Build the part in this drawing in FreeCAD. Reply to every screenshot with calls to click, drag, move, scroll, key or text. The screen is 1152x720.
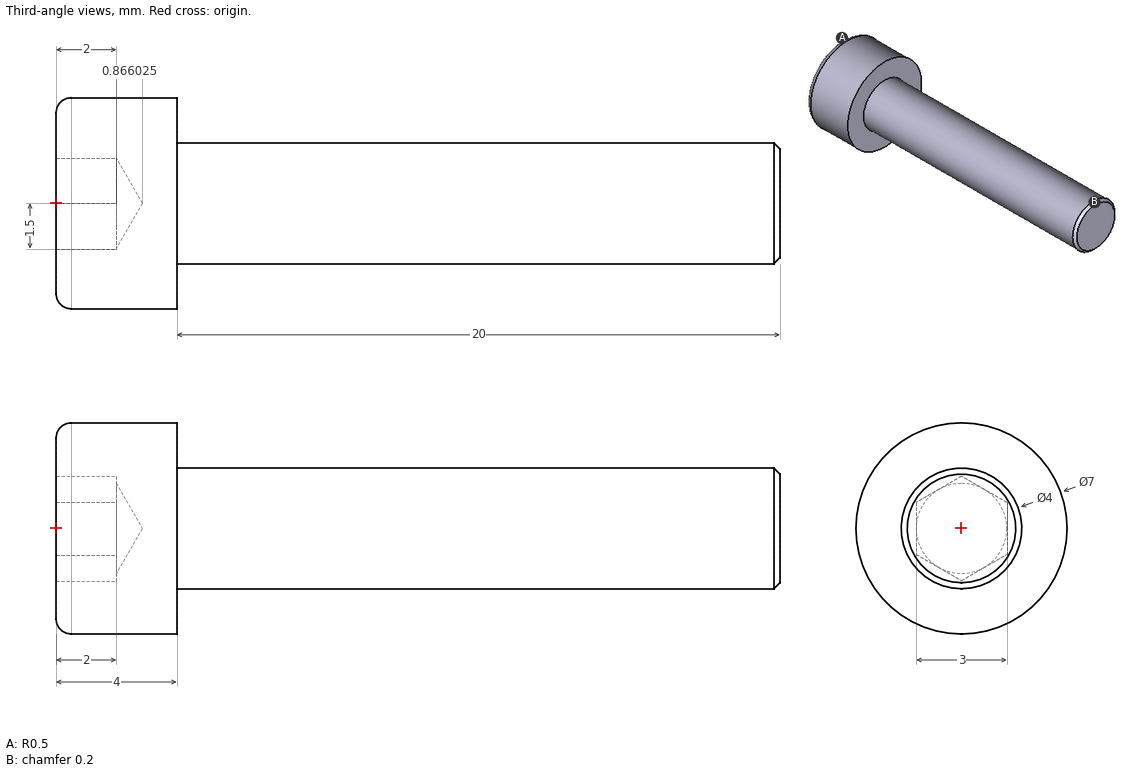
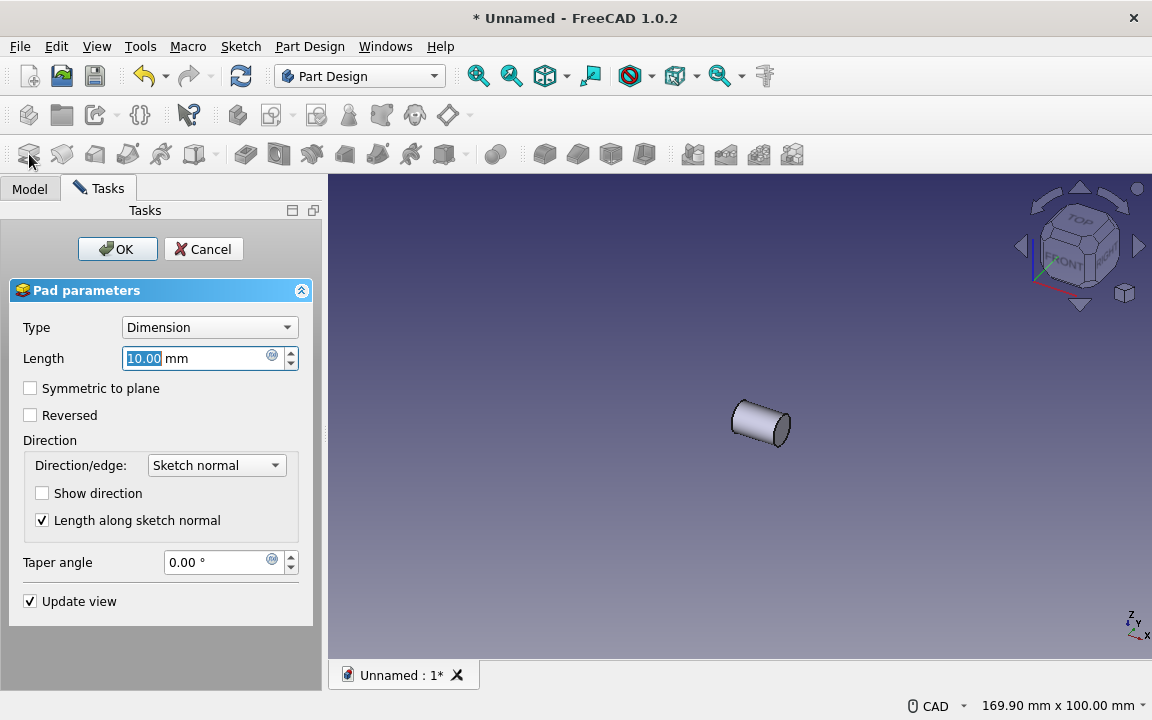
text(4)
key(Tab)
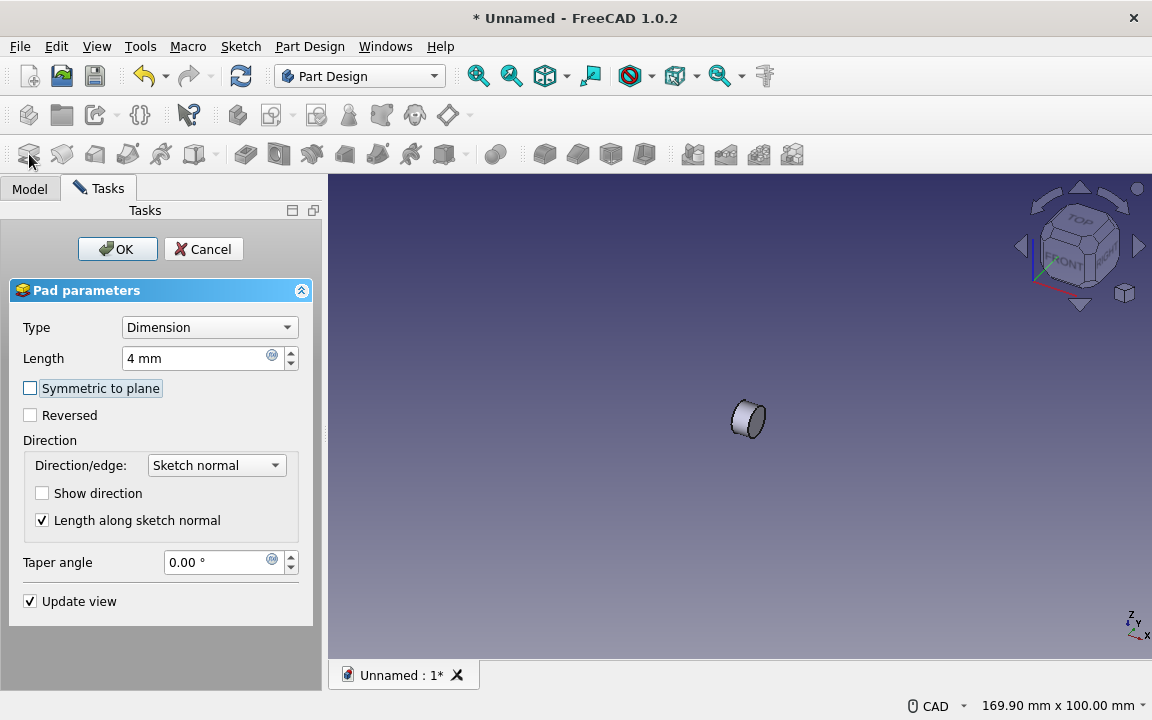
click(118, 249)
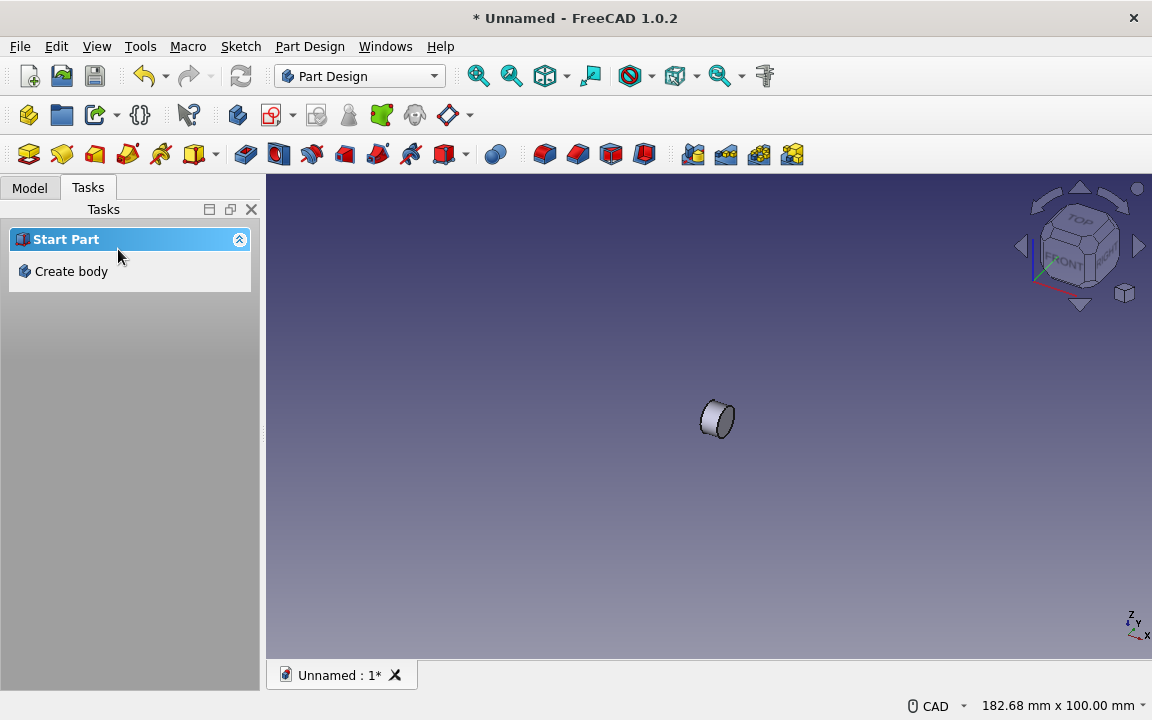
click(479, 76)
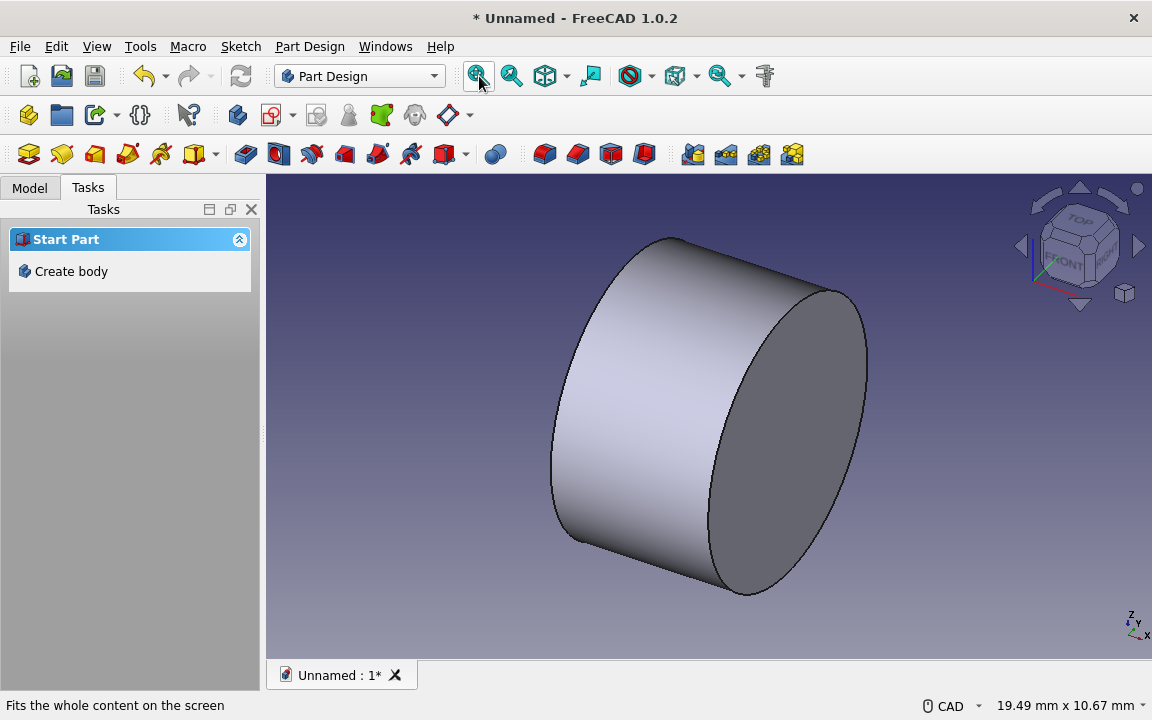
click(788, 442)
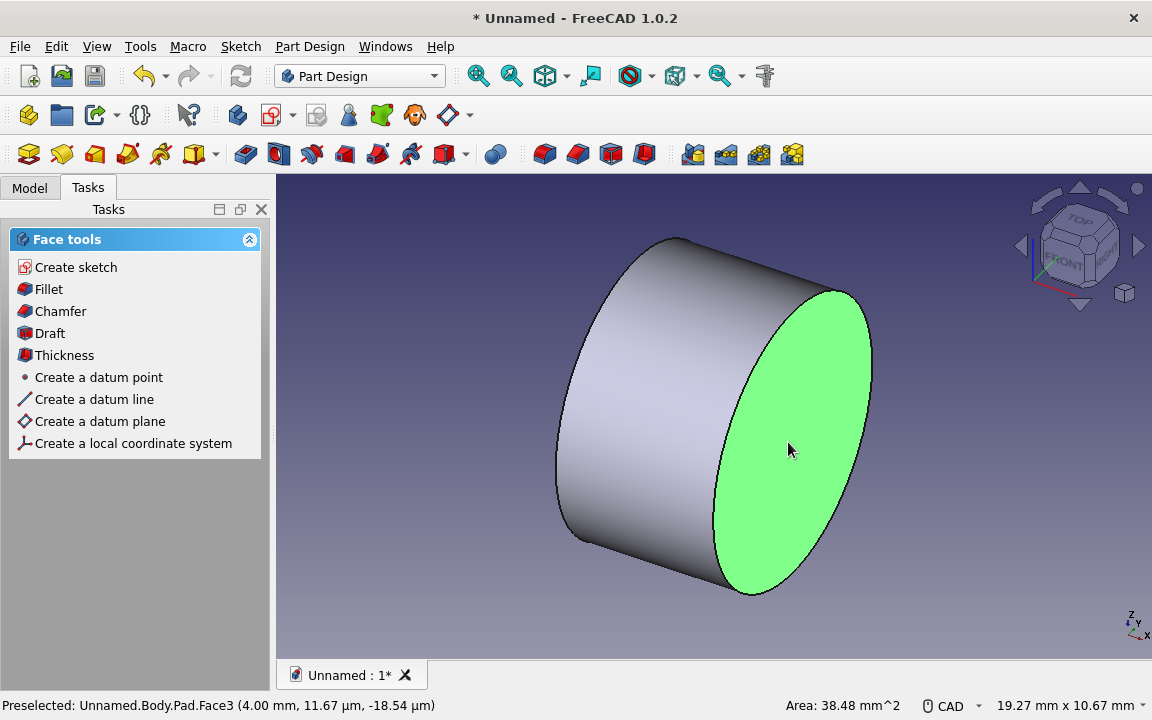
click(270, 116)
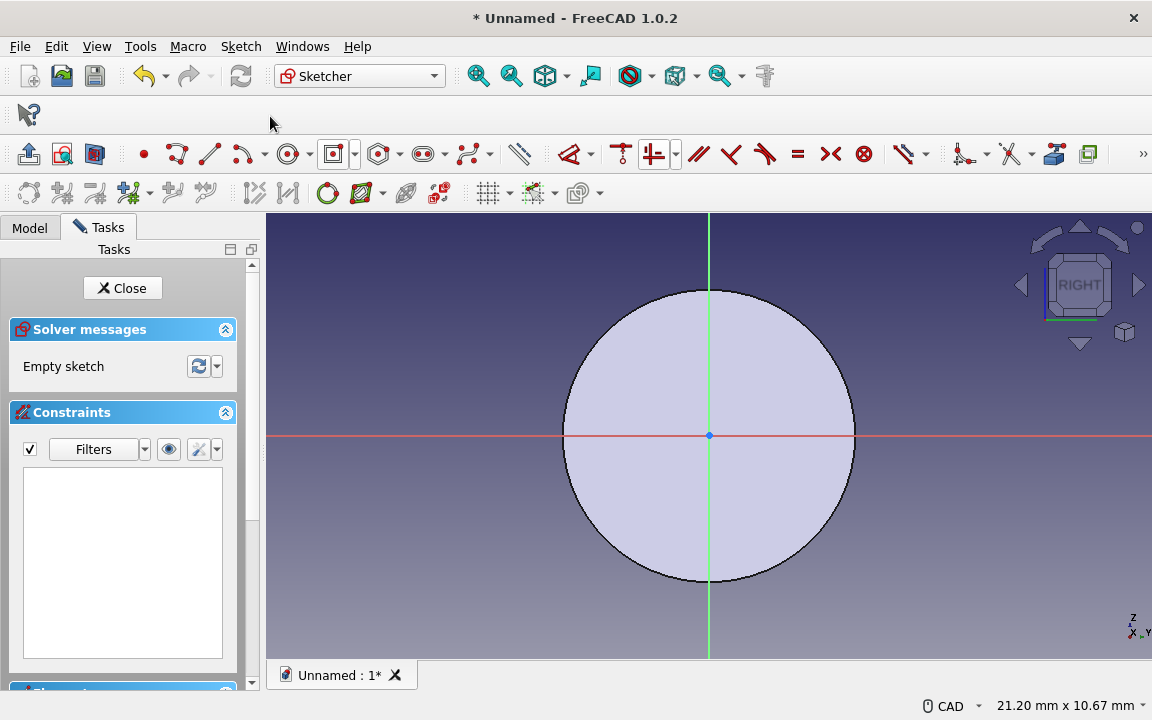
scroll(848, 436, up, 2)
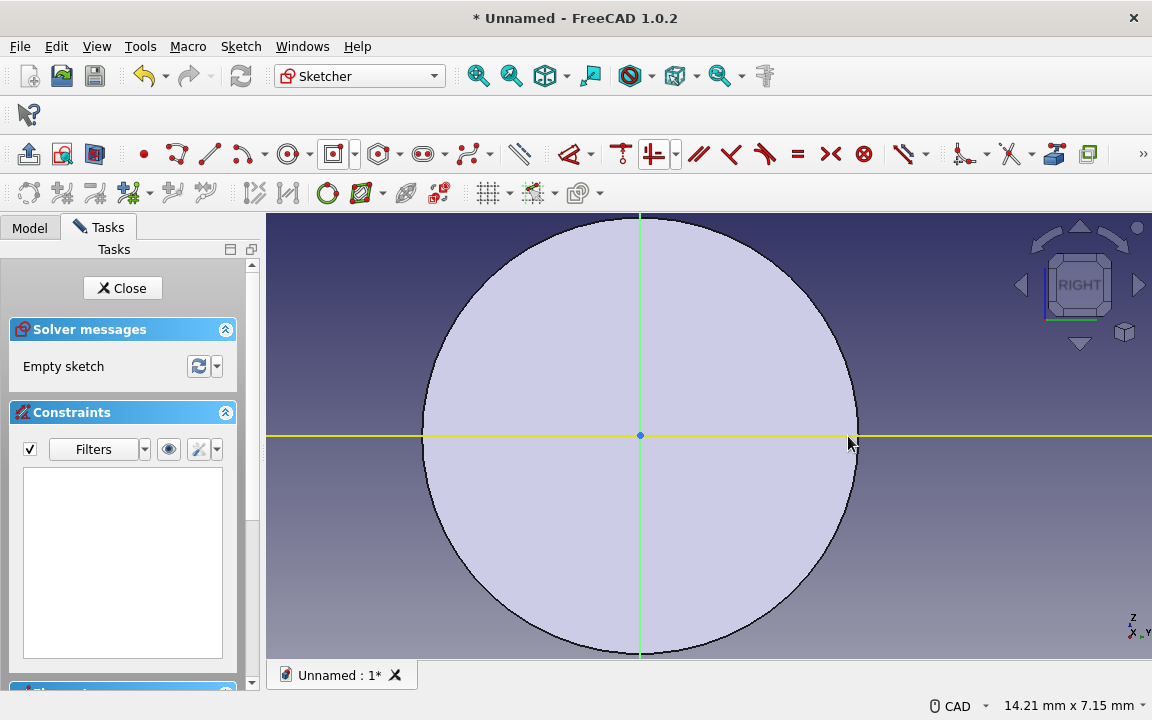
click(288, 154)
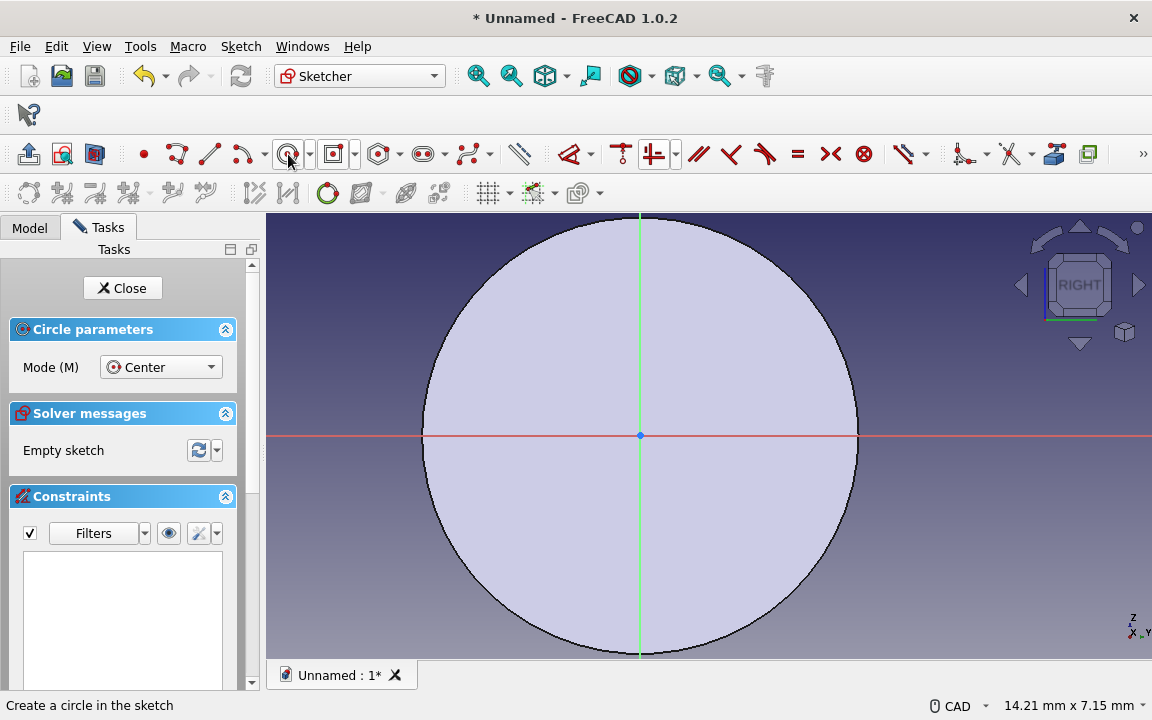
click(640, 436)
click(729, 348)
key(Escape)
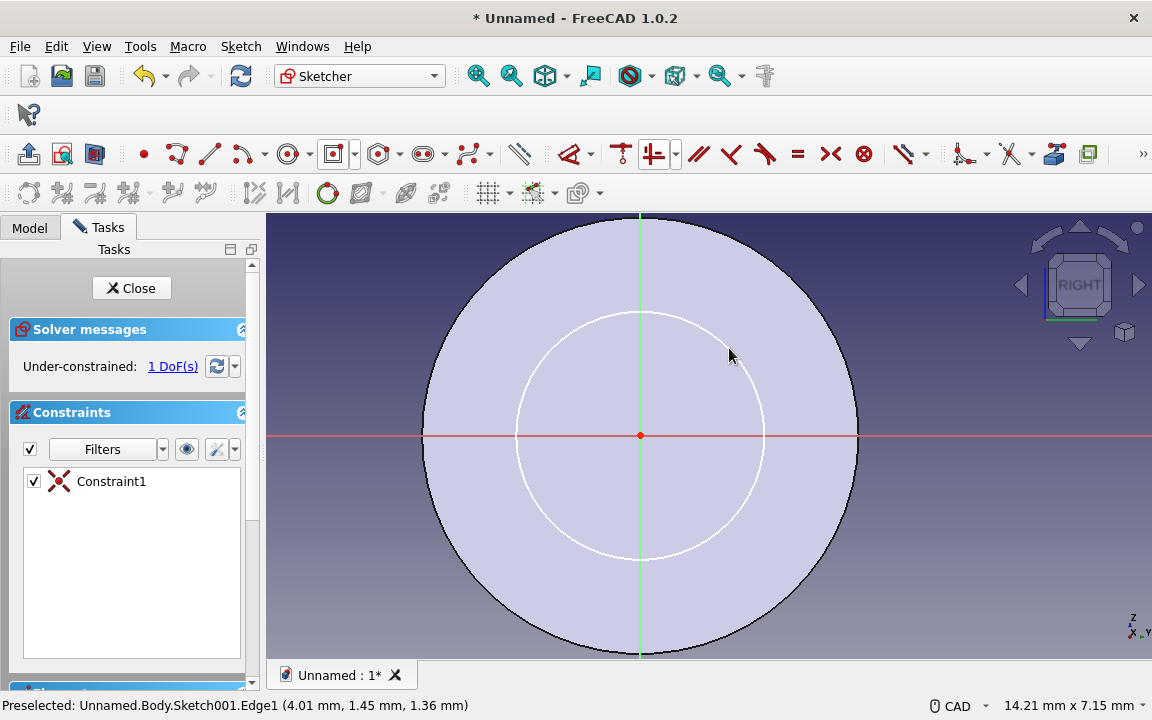
click(568, 154)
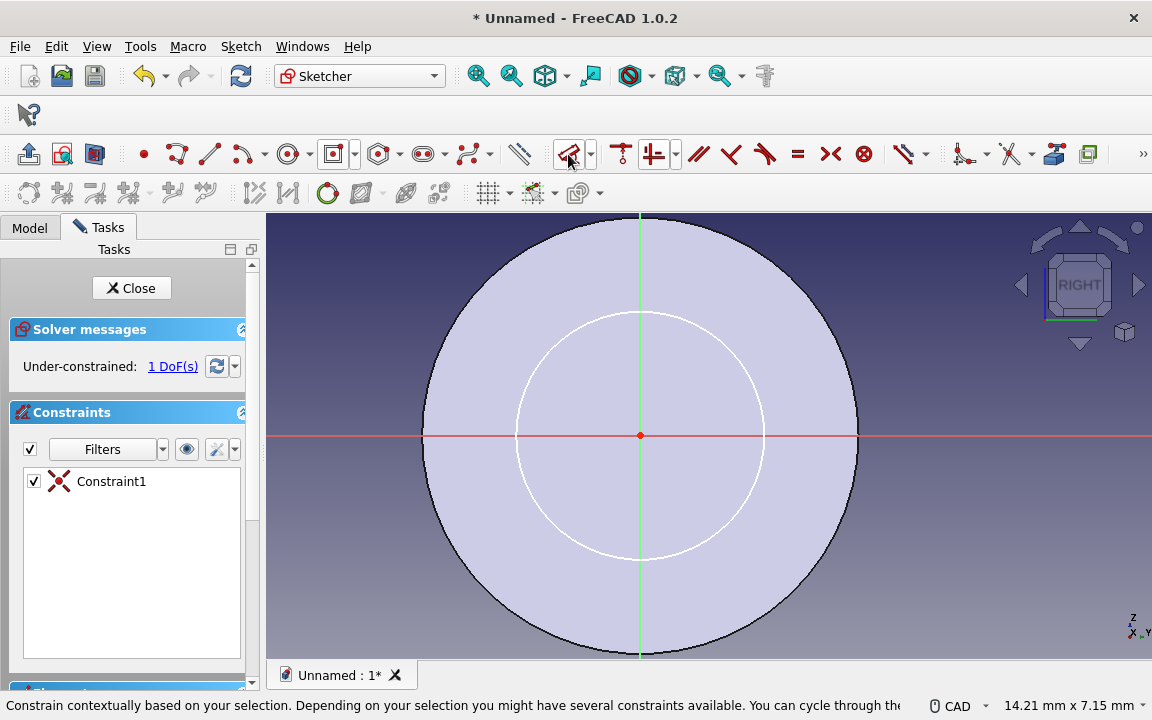
click(728, 348)
click(751, 325)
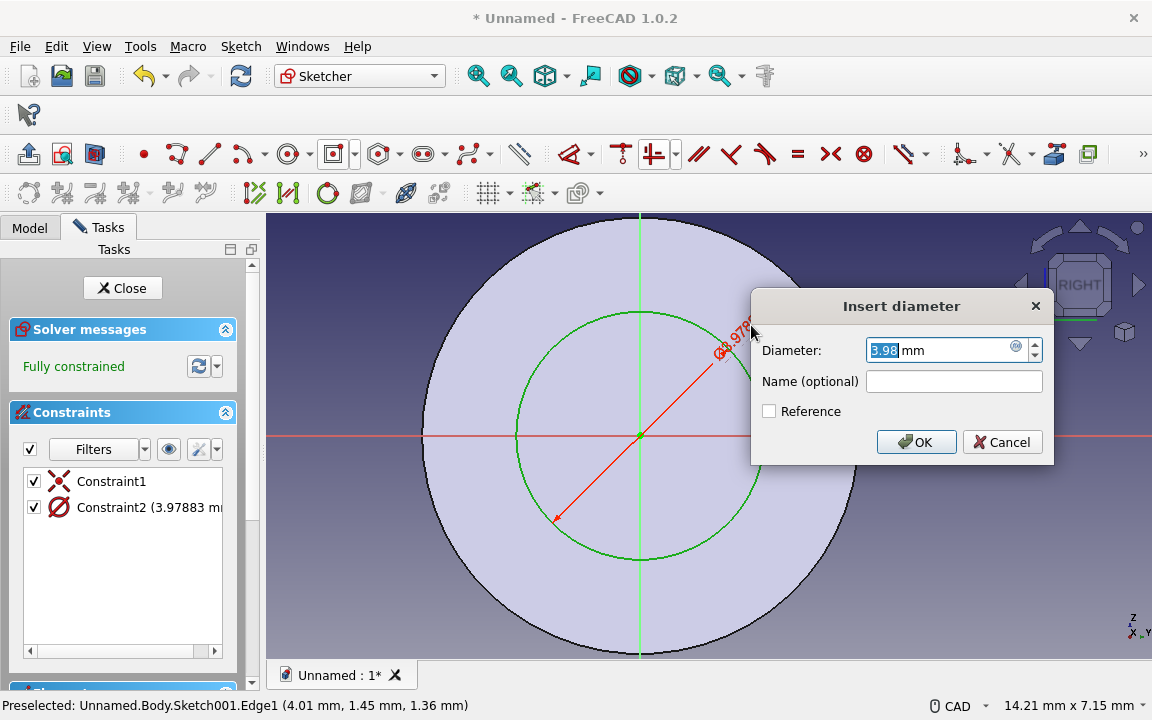
text(4)
key(Return)
key(Escape)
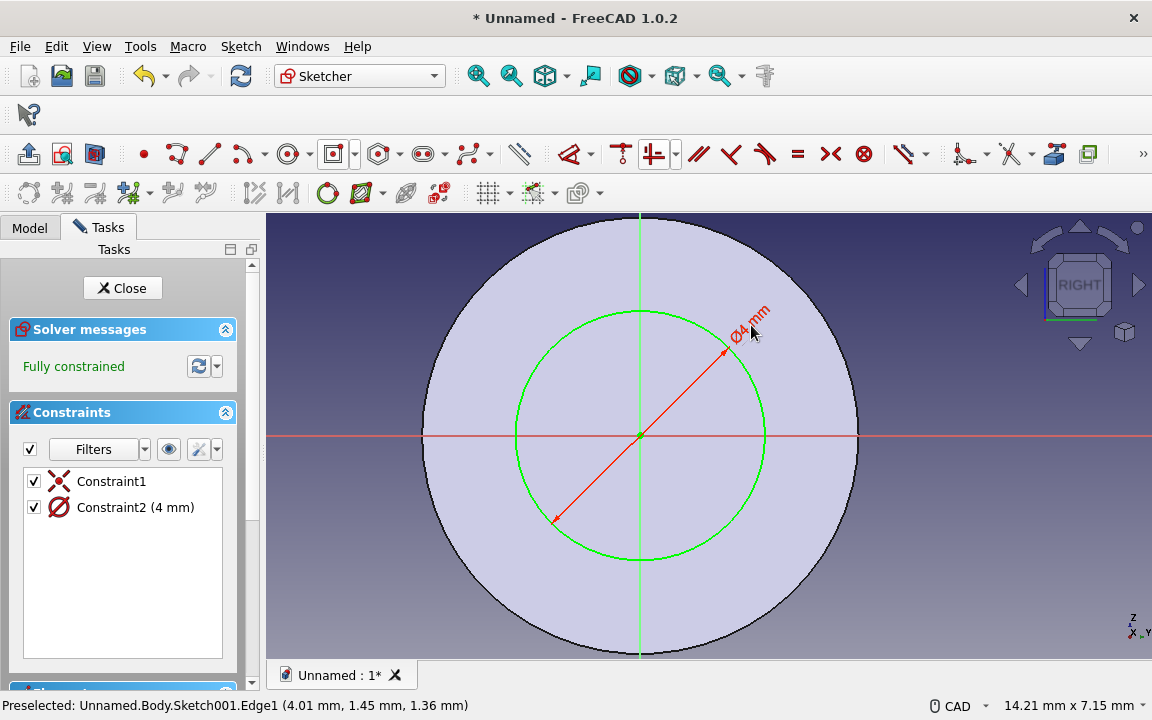
click(123, 288)